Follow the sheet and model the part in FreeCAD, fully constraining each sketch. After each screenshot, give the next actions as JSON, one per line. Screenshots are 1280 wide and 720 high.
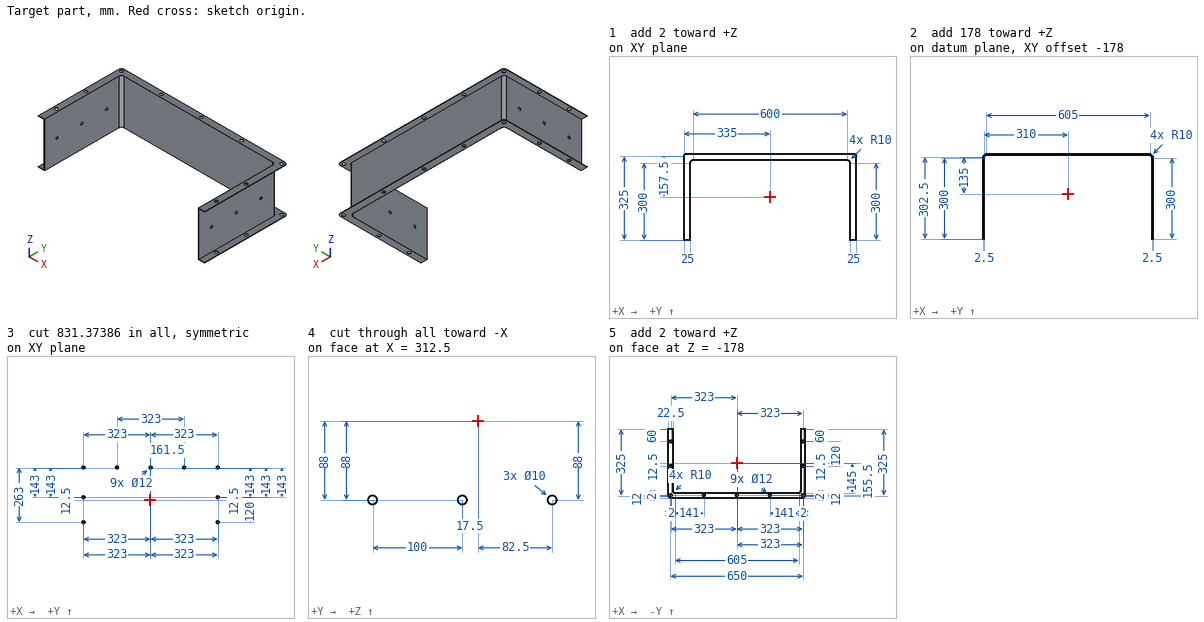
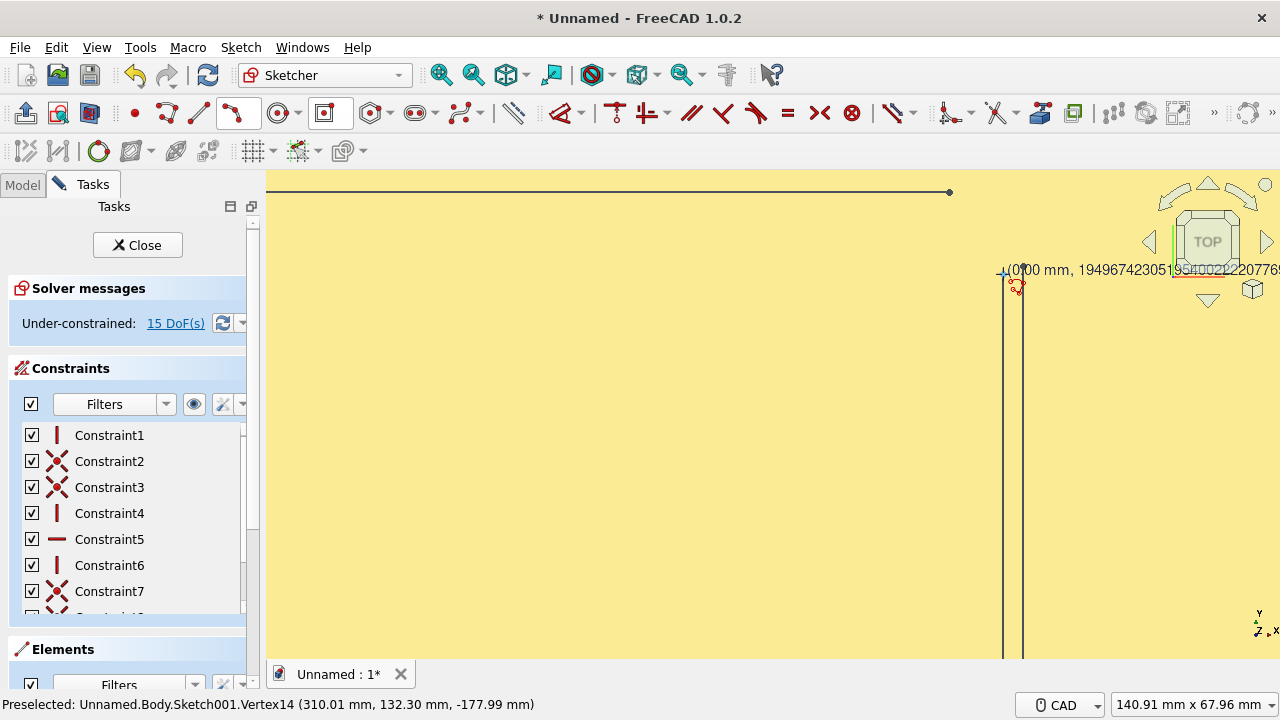
{"action": "key", "text": "g l"}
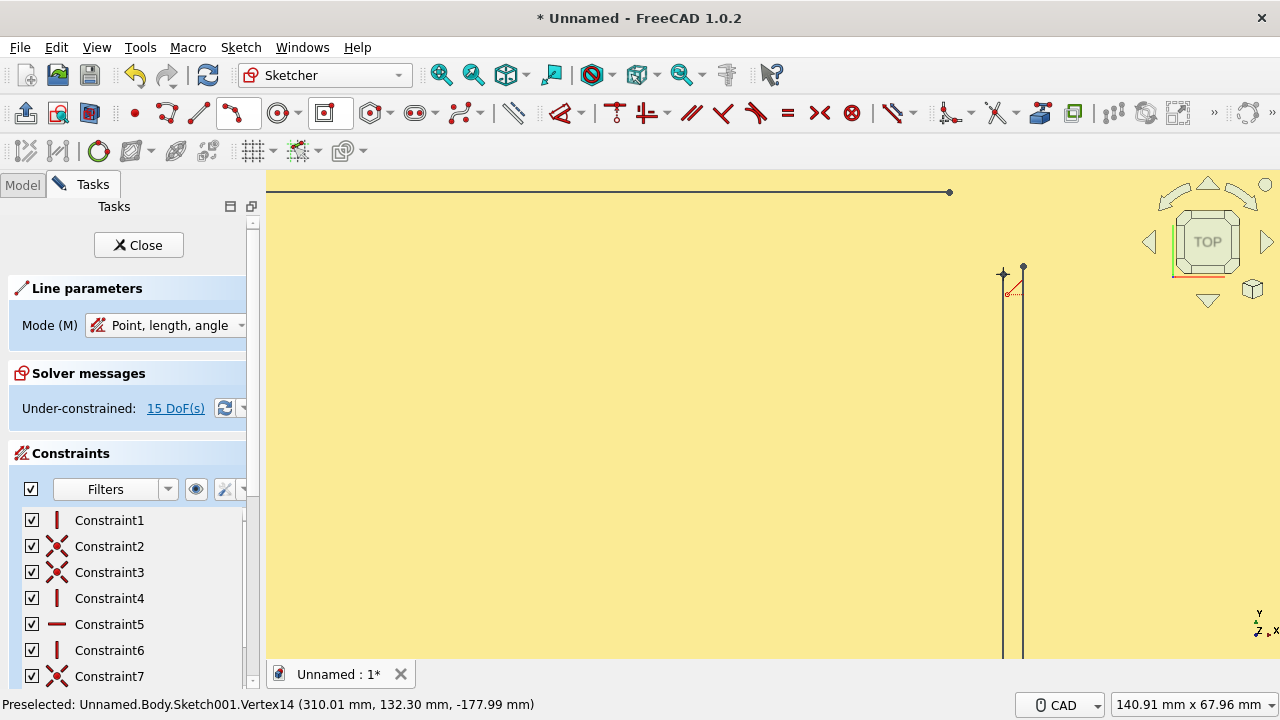
{"action": "left_click", "coordinate": [931, 202]}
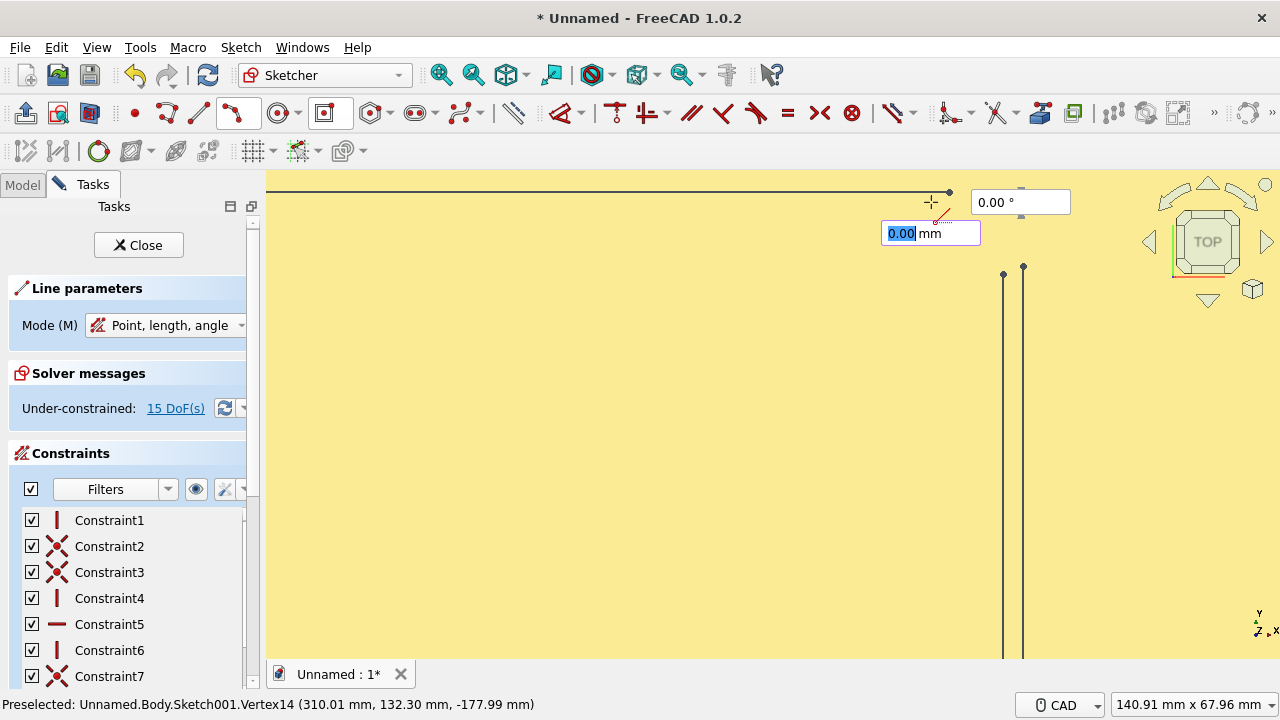
{"action": "scroll", "coordinate": [1007, 275], "scroll_direction": "down", "scroll_amount": 10}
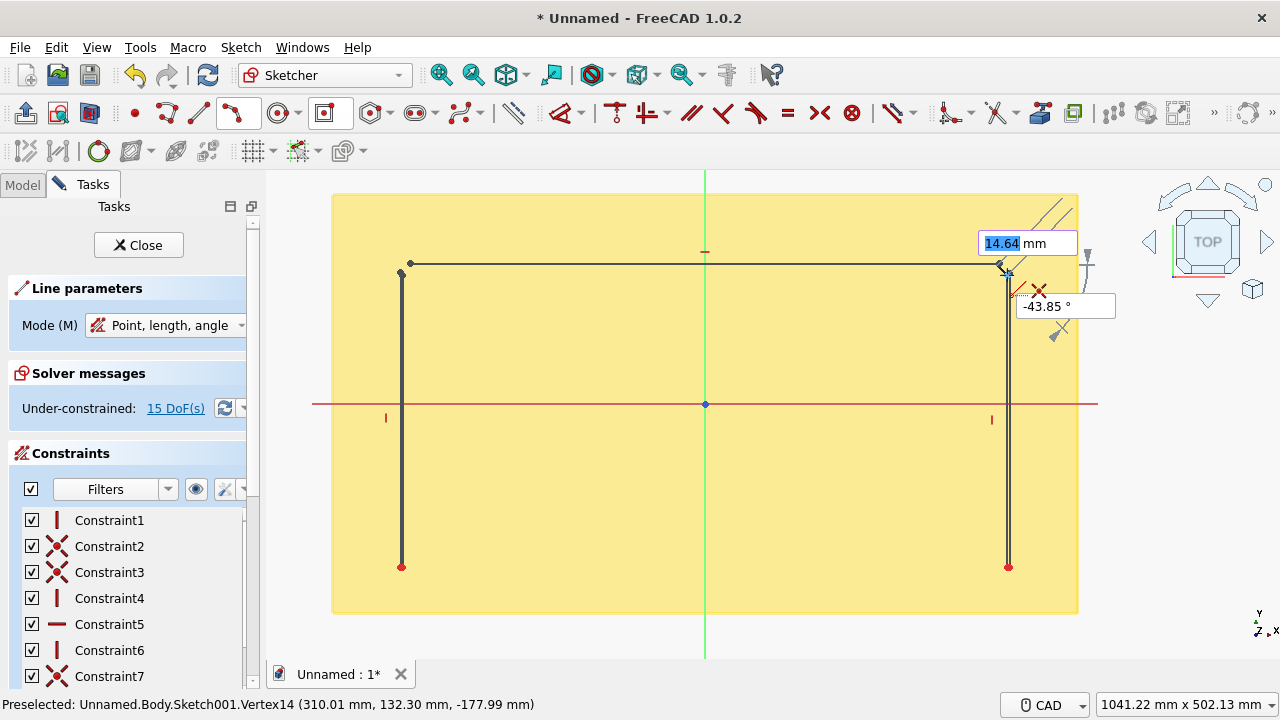
{"action": "scroll", "coordinate": [413, 265], "scroll_direction": "up", "scroll_amount": 10}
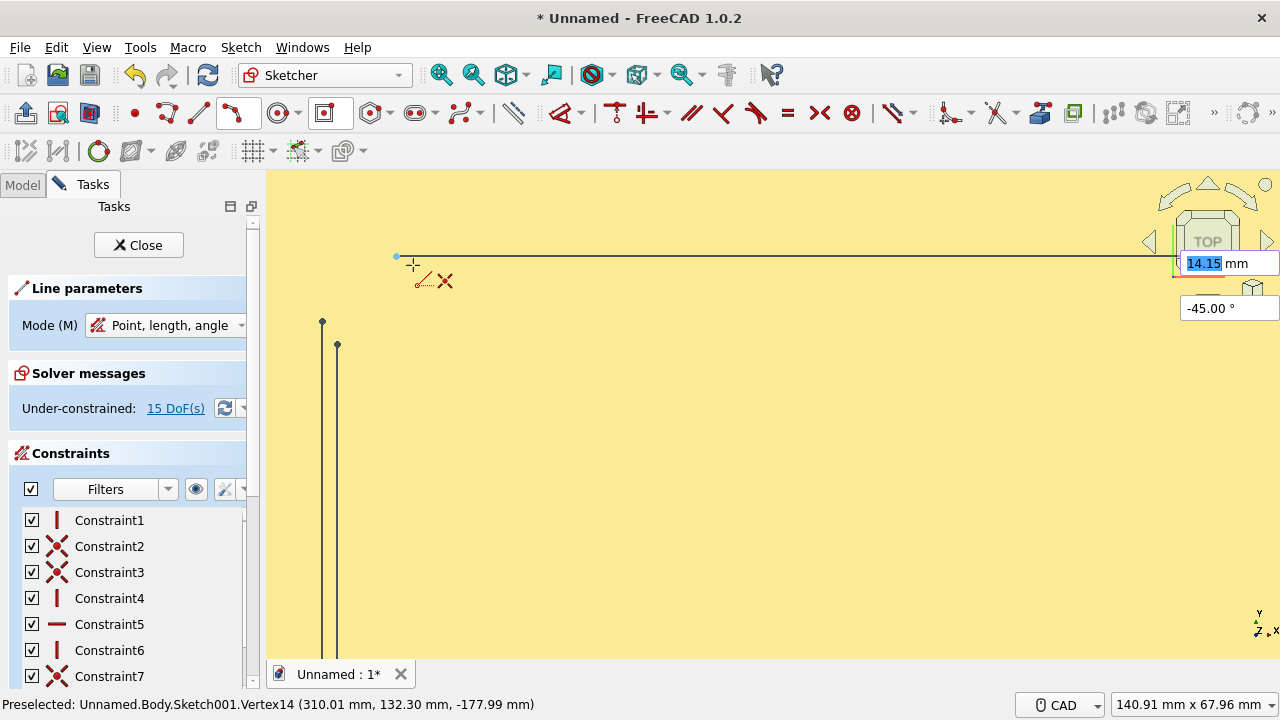
{"action": "left_click", "coordinate": [412, 266]}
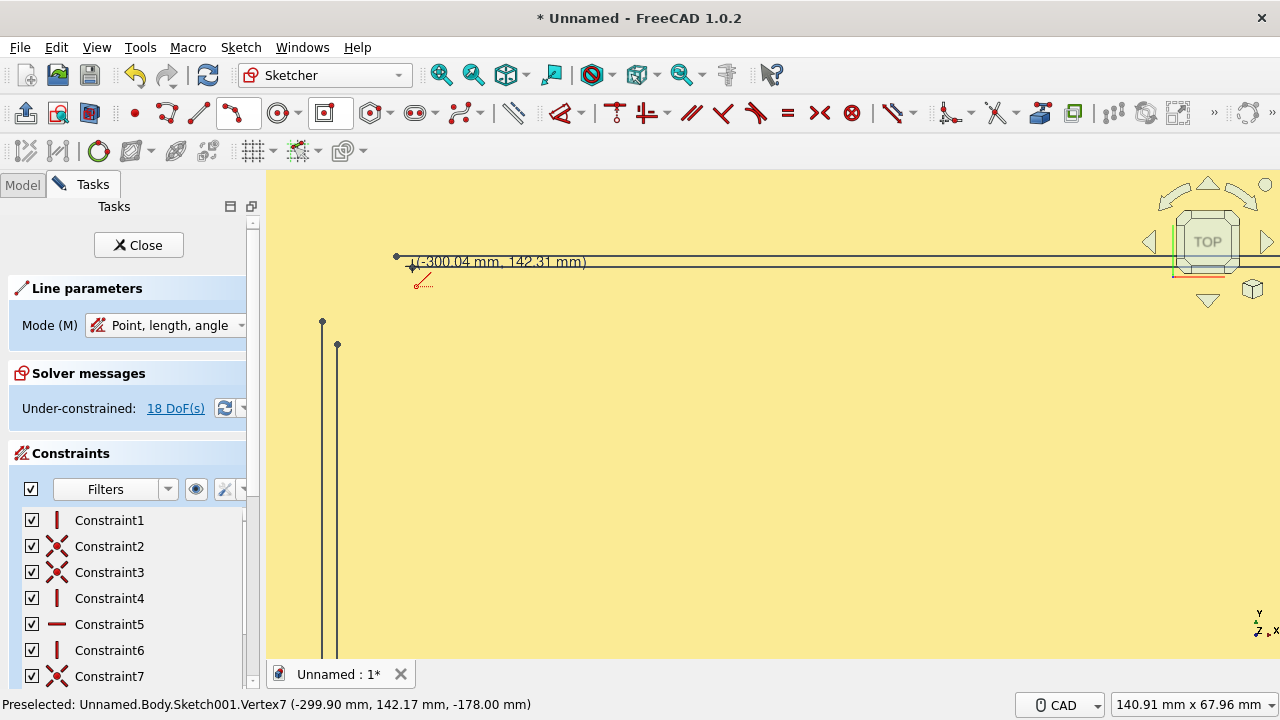
{"action": "left_click", "coordinate": [232, 114]}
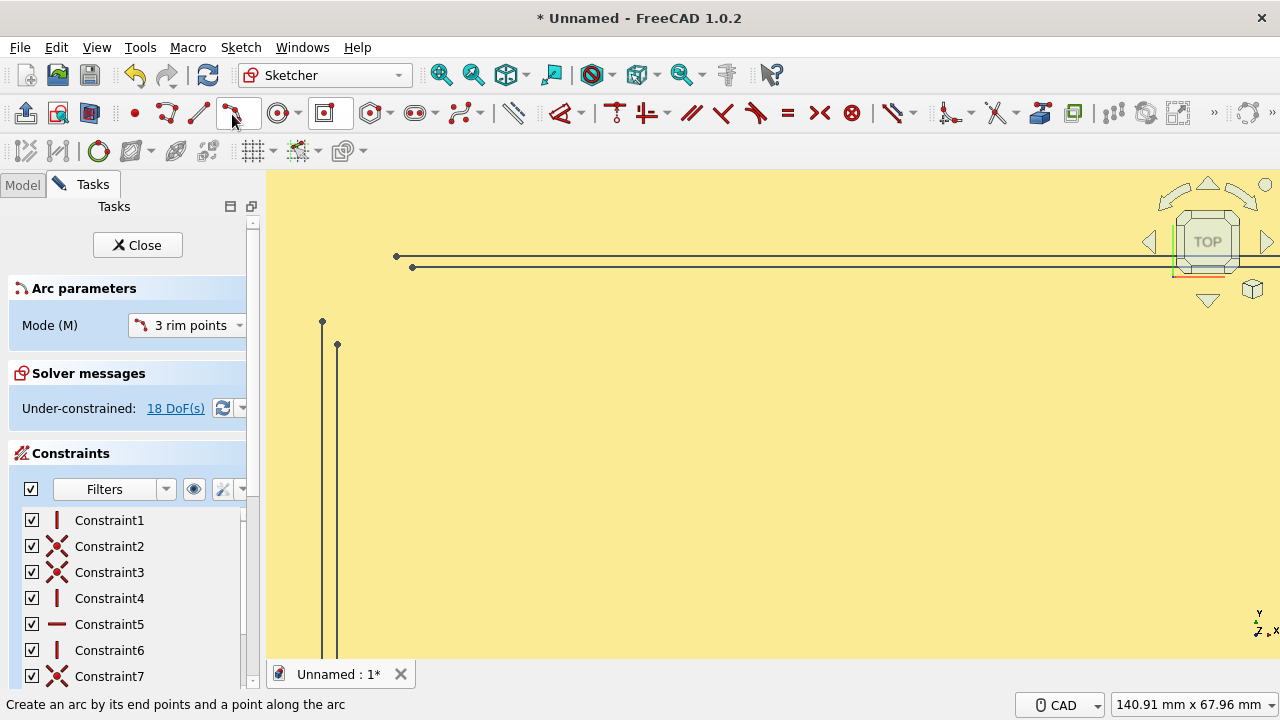
{"action": "left_click", "coordinate": [322, 321]}
{"action": "left_click", "coordinate": [396, 256]}
{"action": "left_click", "coordinate": [343, 269]}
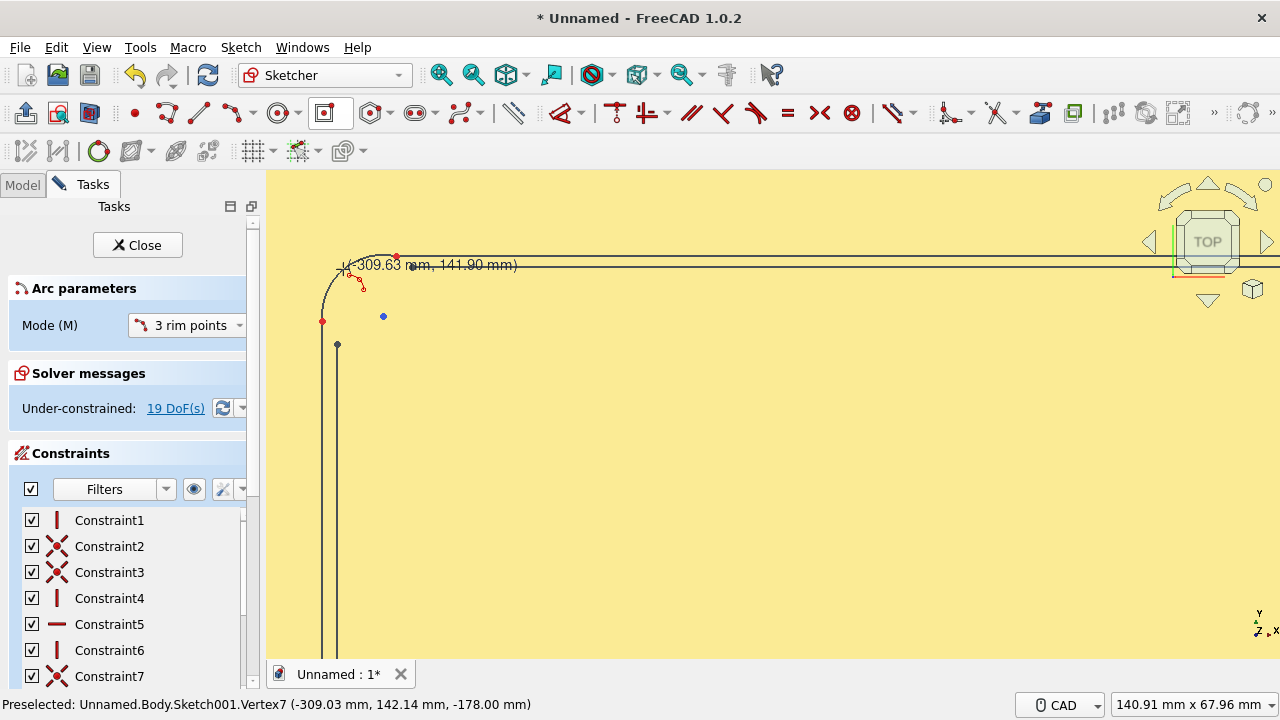
{"action": "scroll", "coordinate": [412, 265], "scroll_direction": "down", "scroll_amount": 10}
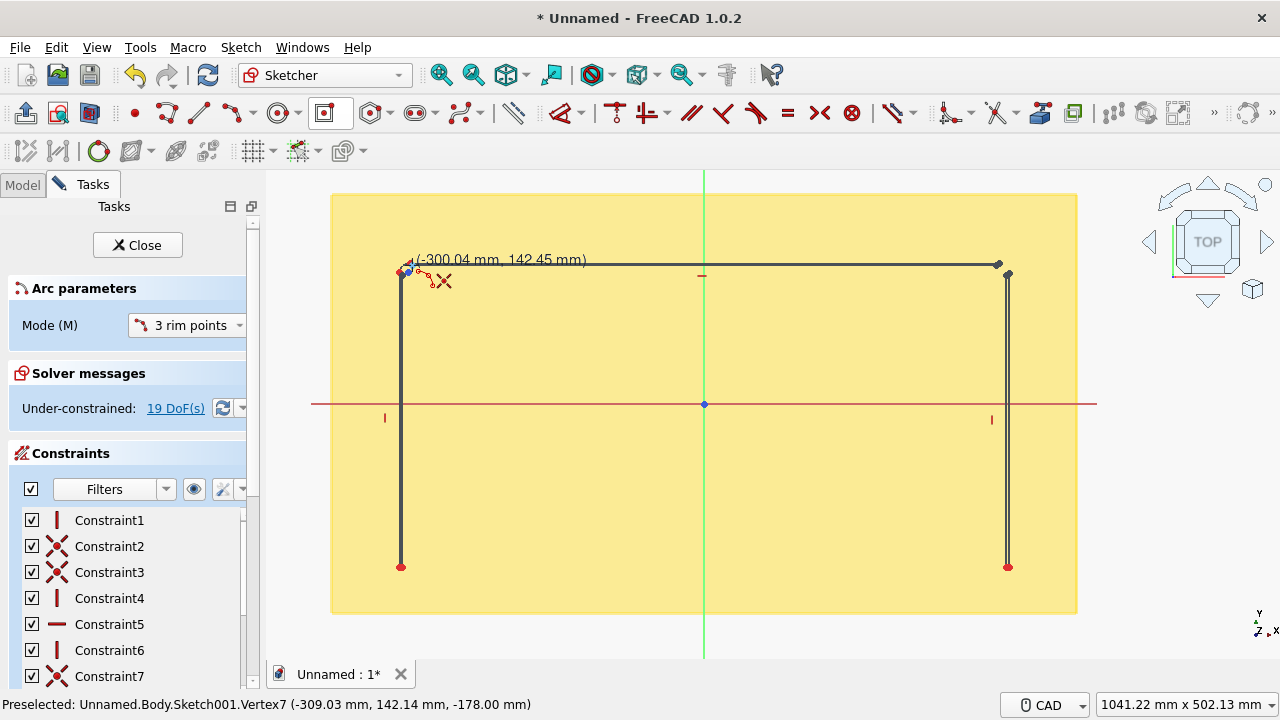
{"action": "scroll", "coordinate": [999, 263], "scroll_direction": "up", "scroll_amount": 8}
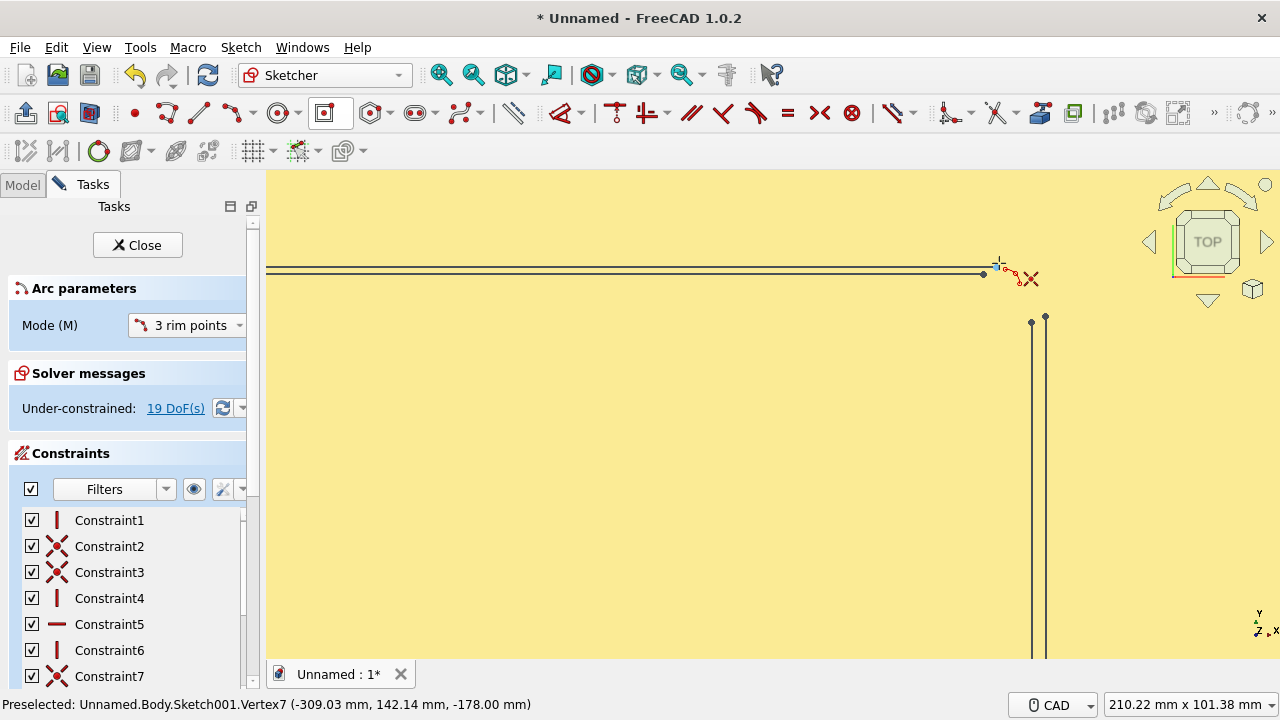
{"action": "left_click", "coordinate": [996, 267]}
{"action": "left_click", "coordinate": [1046, 317]}
{"action": "left_click", "coordinate": [1030, 275]}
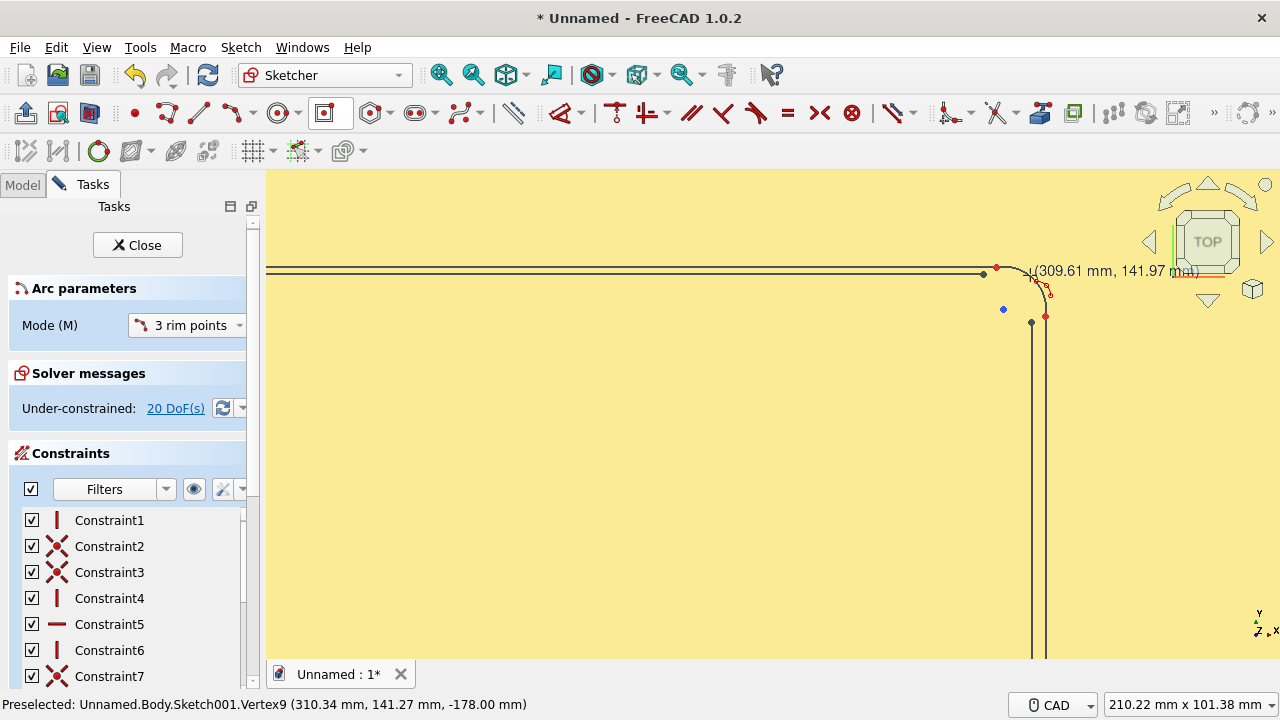
{"action": "scroll", "coordinate": [1032, 322], "scroll_direction": "up", "scroll_amount": 2}